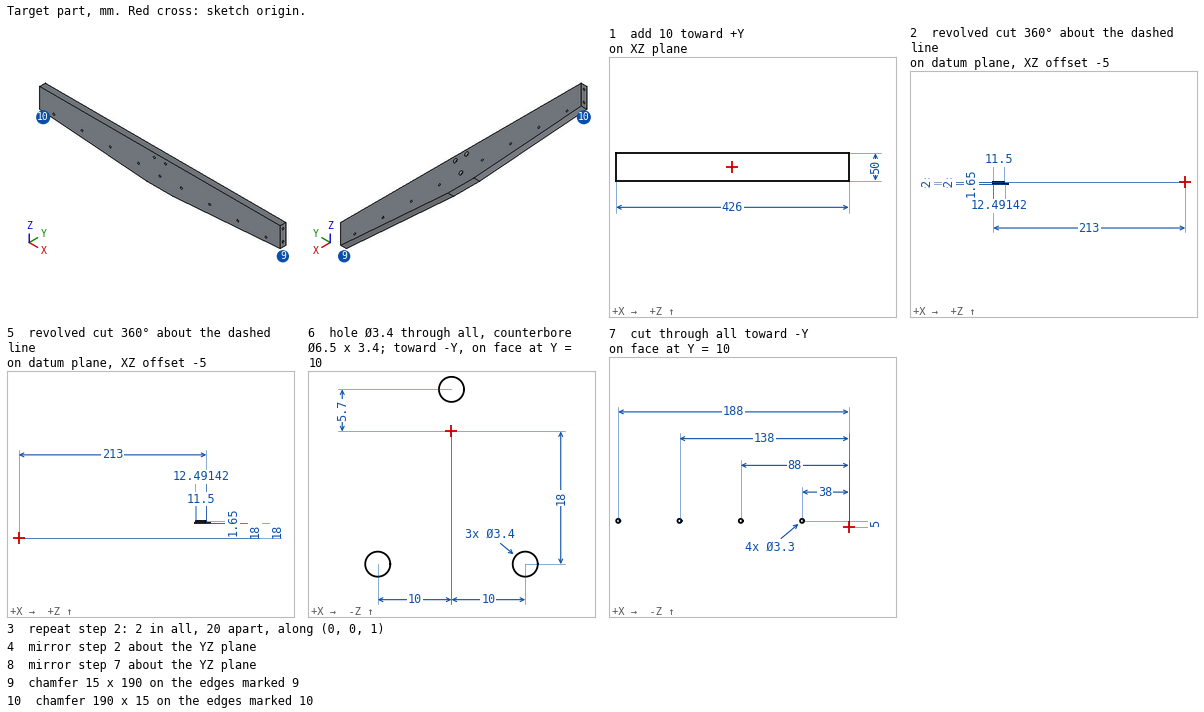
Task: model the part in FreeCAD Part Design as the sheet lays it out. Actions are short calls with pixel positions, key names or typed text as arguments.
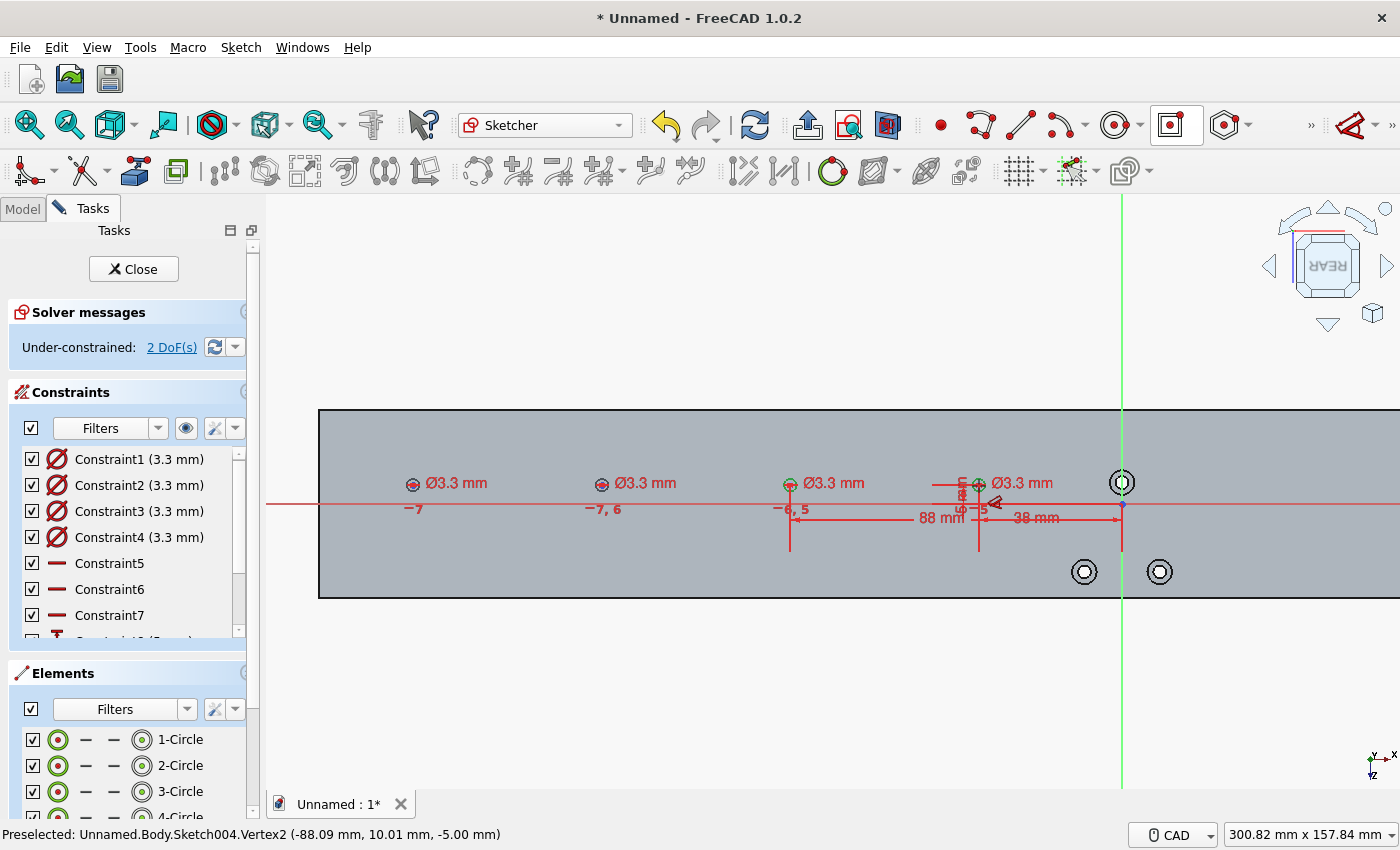
click(602, 485)
click(862, 538)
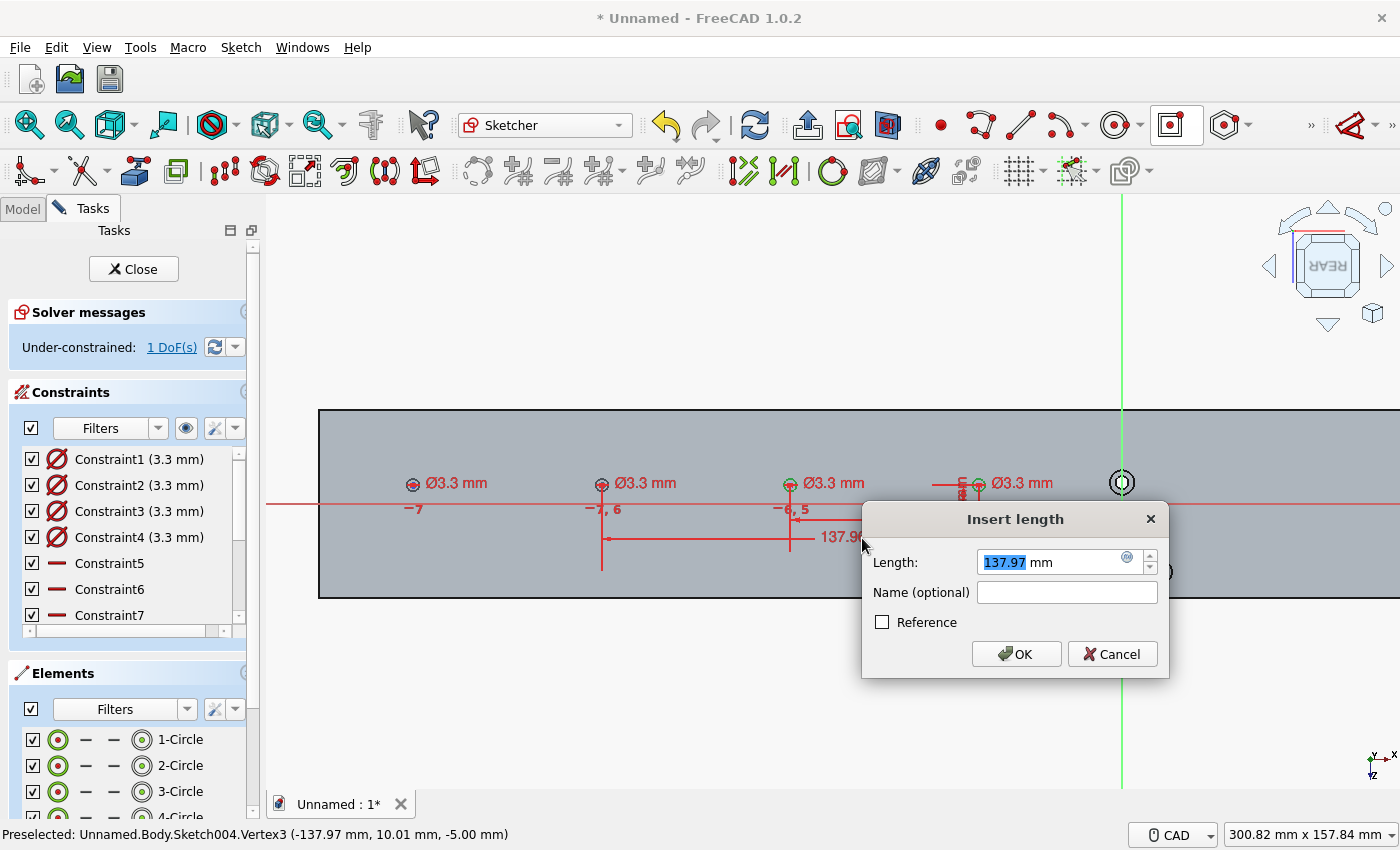
text(138)
key(Return)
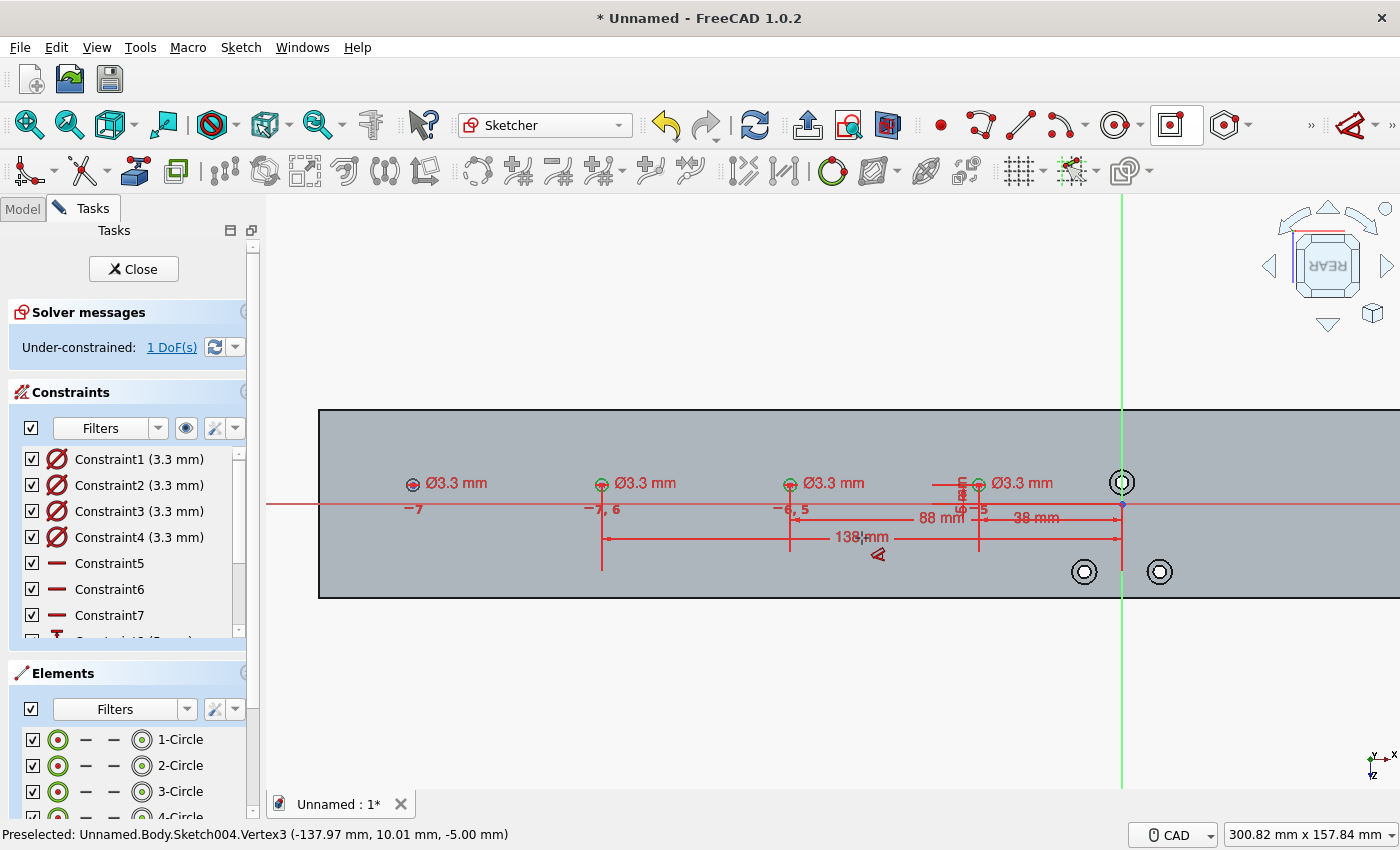
click(413, 485)
click(768, 538)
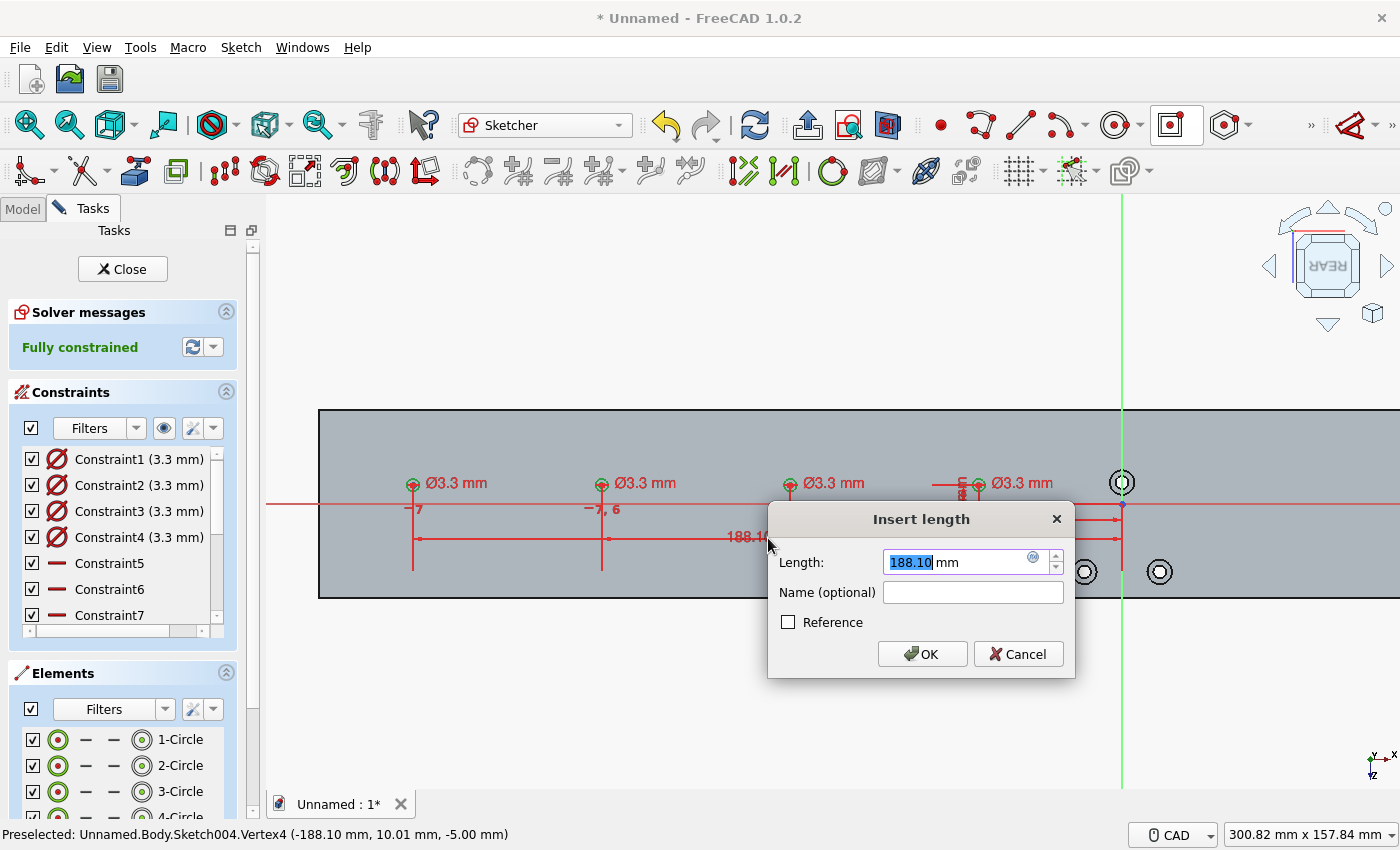
text(188)
key(Return)
key(Escape)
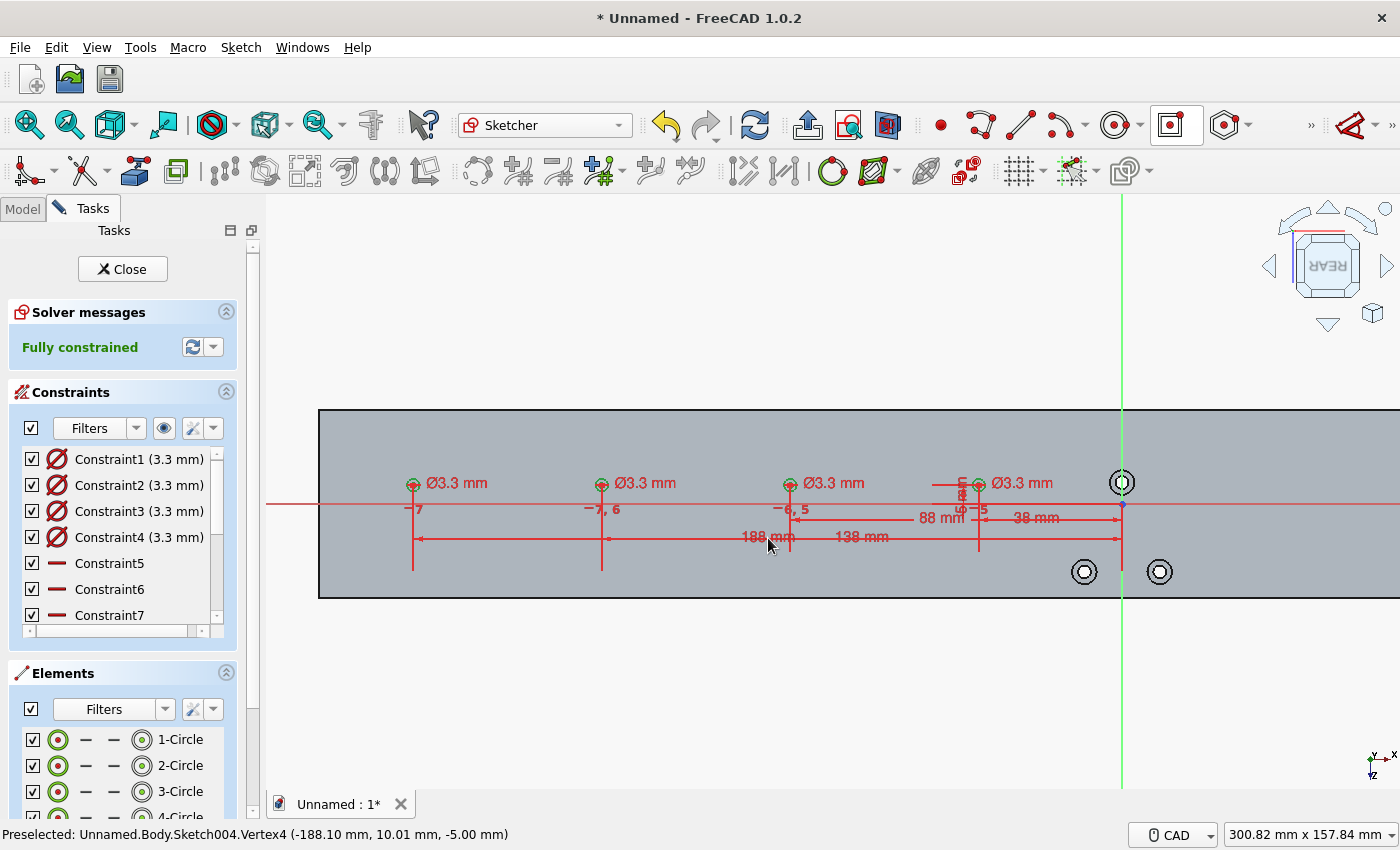
click(123, 269)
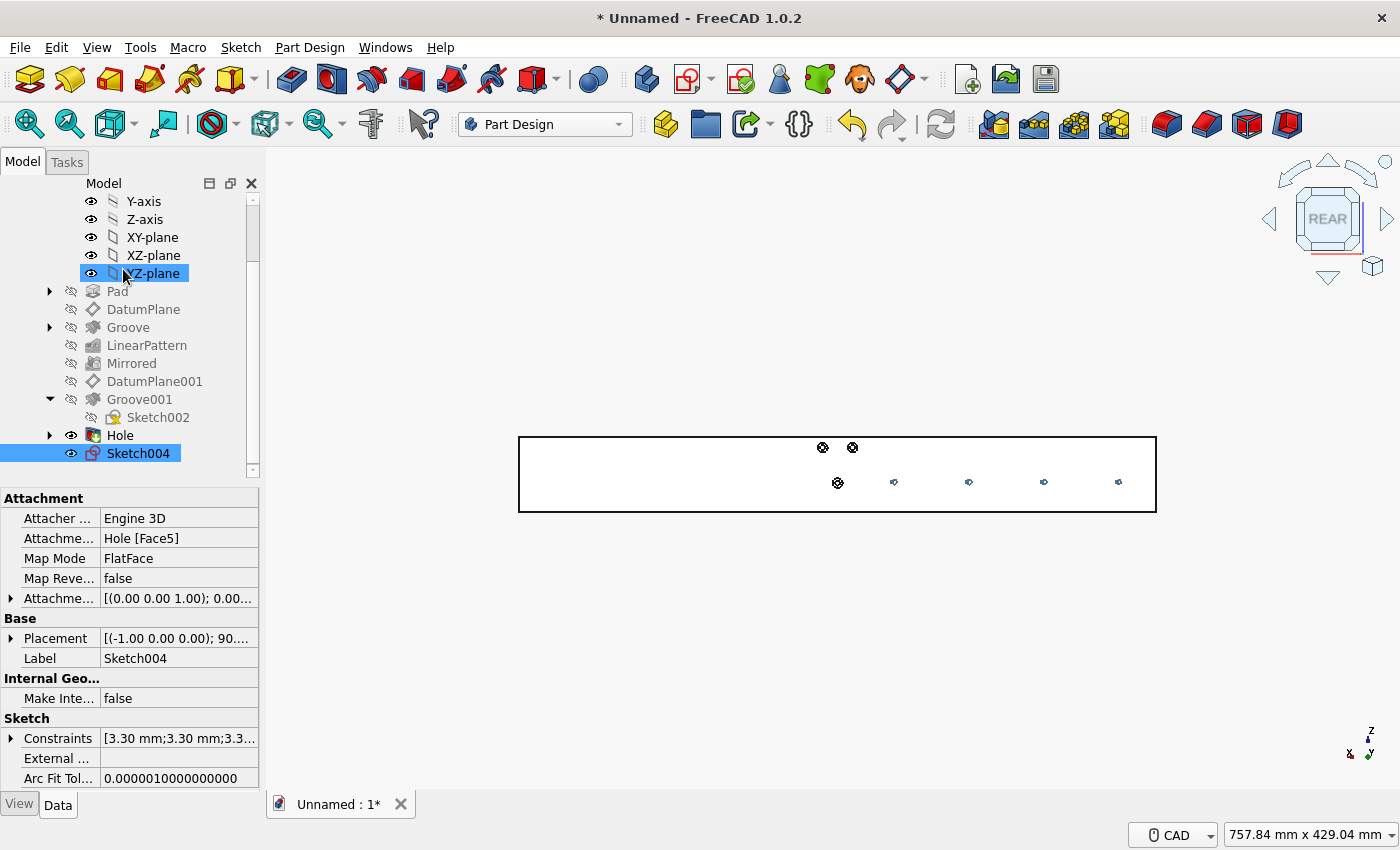
click(292, 80)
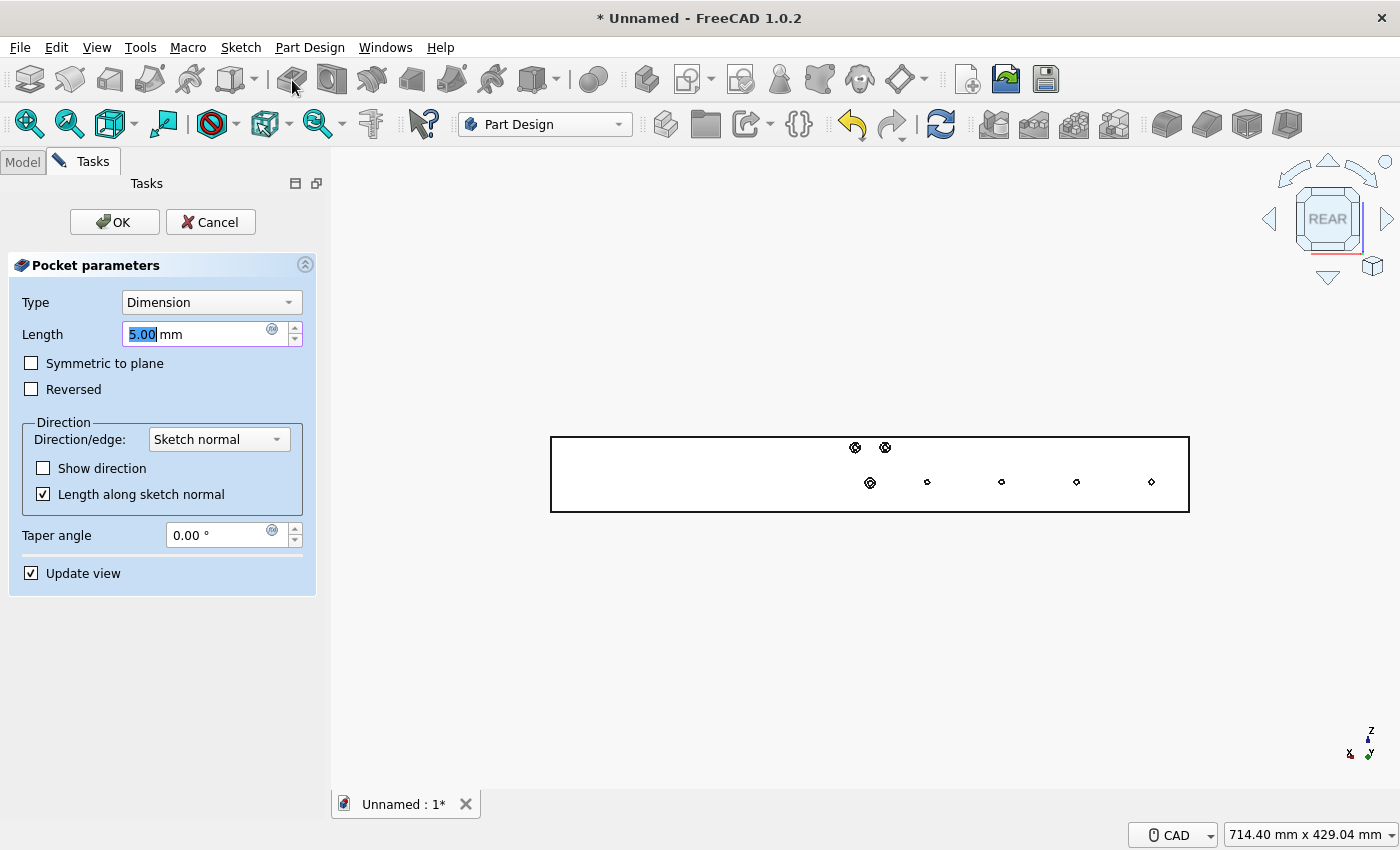
click(212, 302)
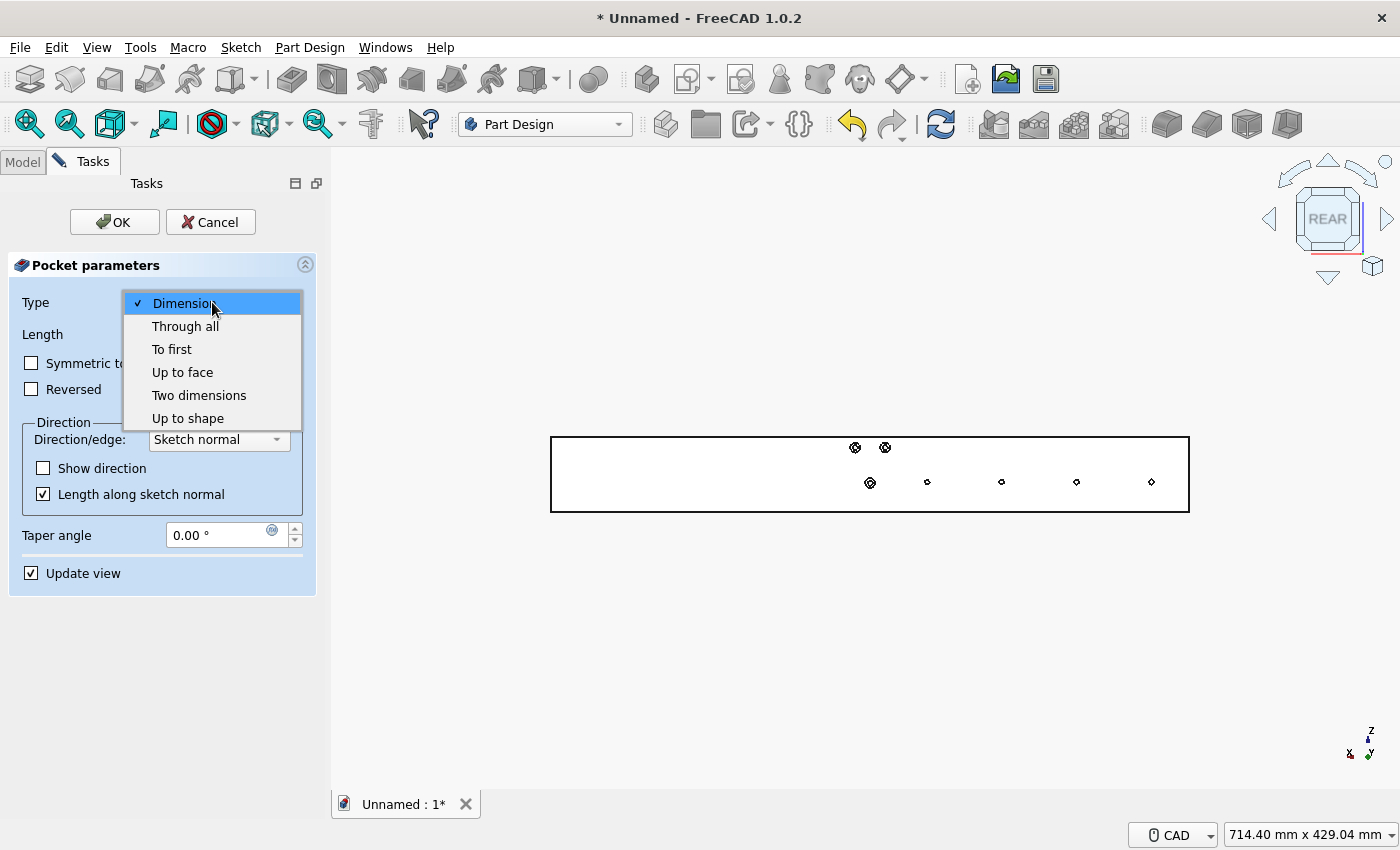
click(212, 326)